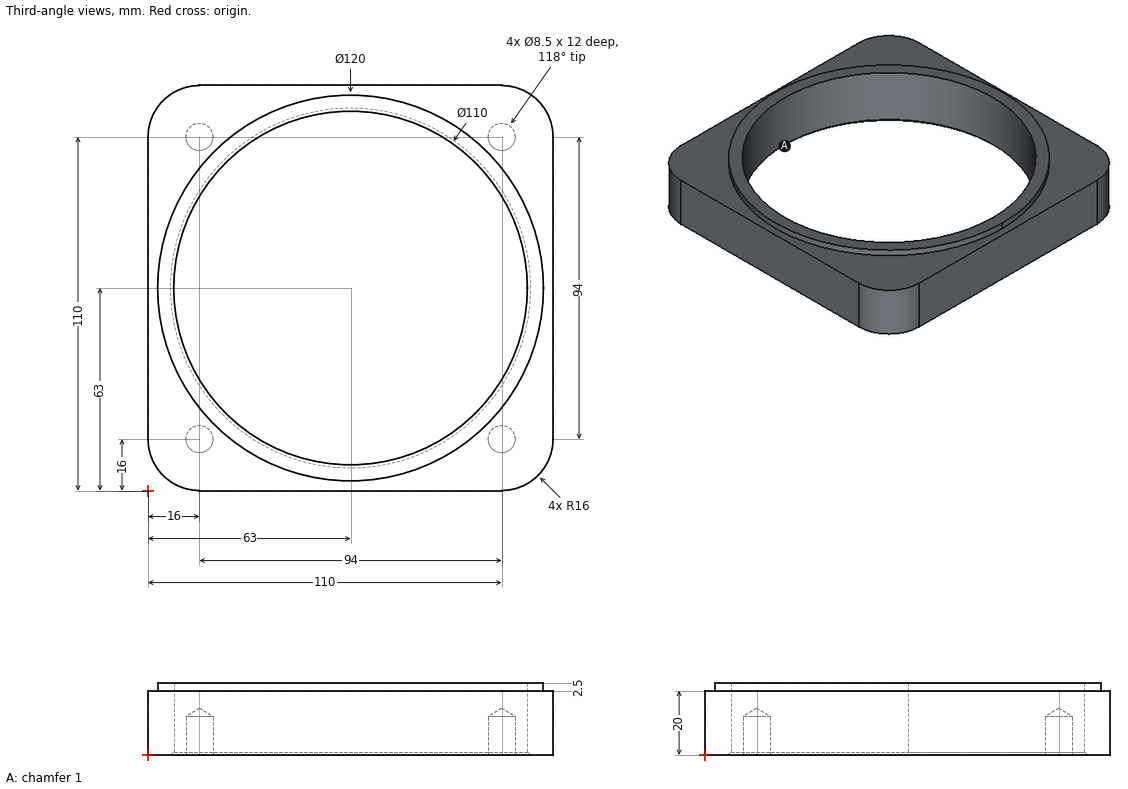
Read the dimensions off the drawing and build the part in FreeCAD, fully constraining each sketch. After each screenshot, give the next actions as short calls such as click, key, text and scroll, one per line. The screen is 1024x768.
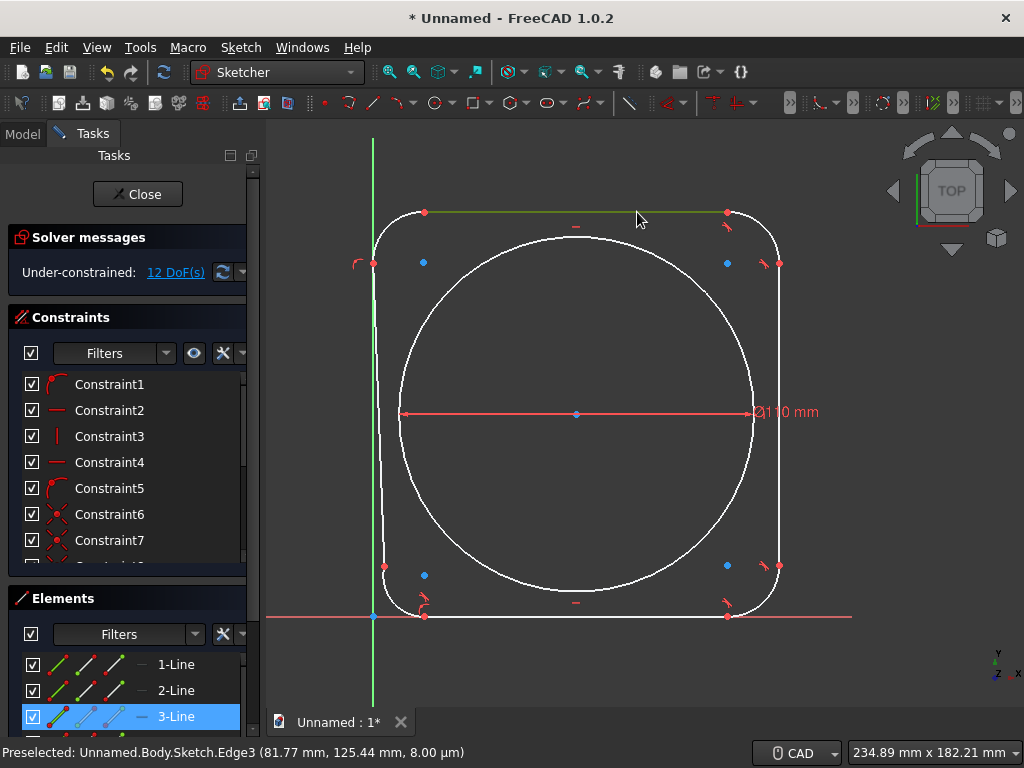
click(401, 217)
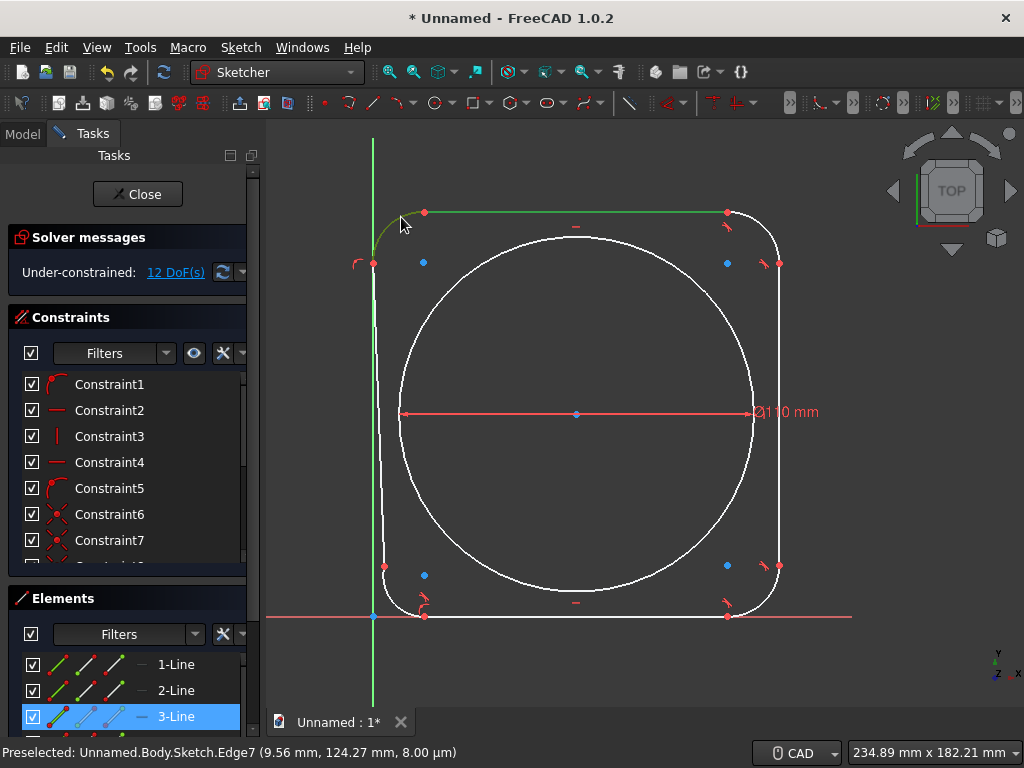
key(t)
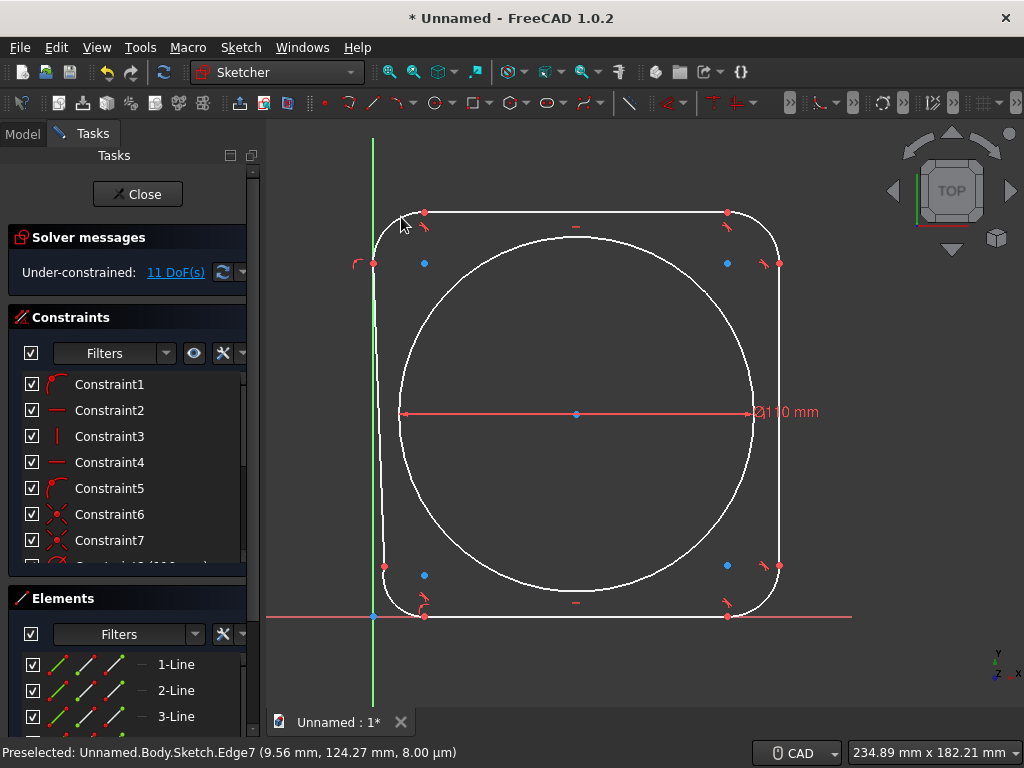
click(377, 354)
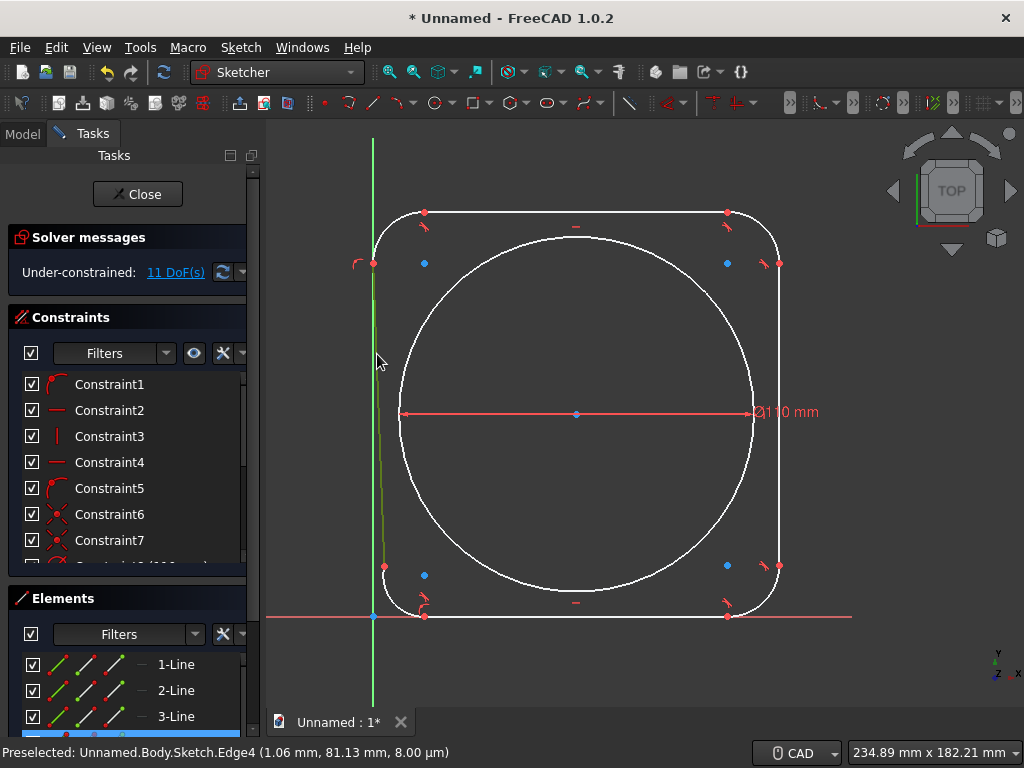
click(401, 218)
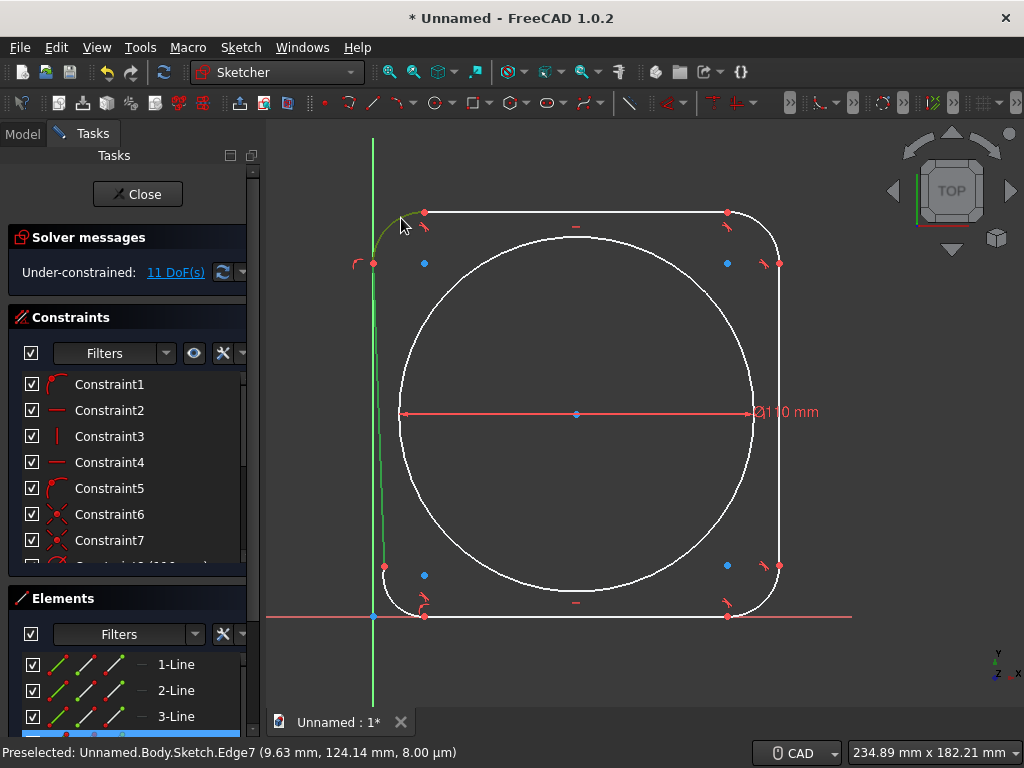
key(t)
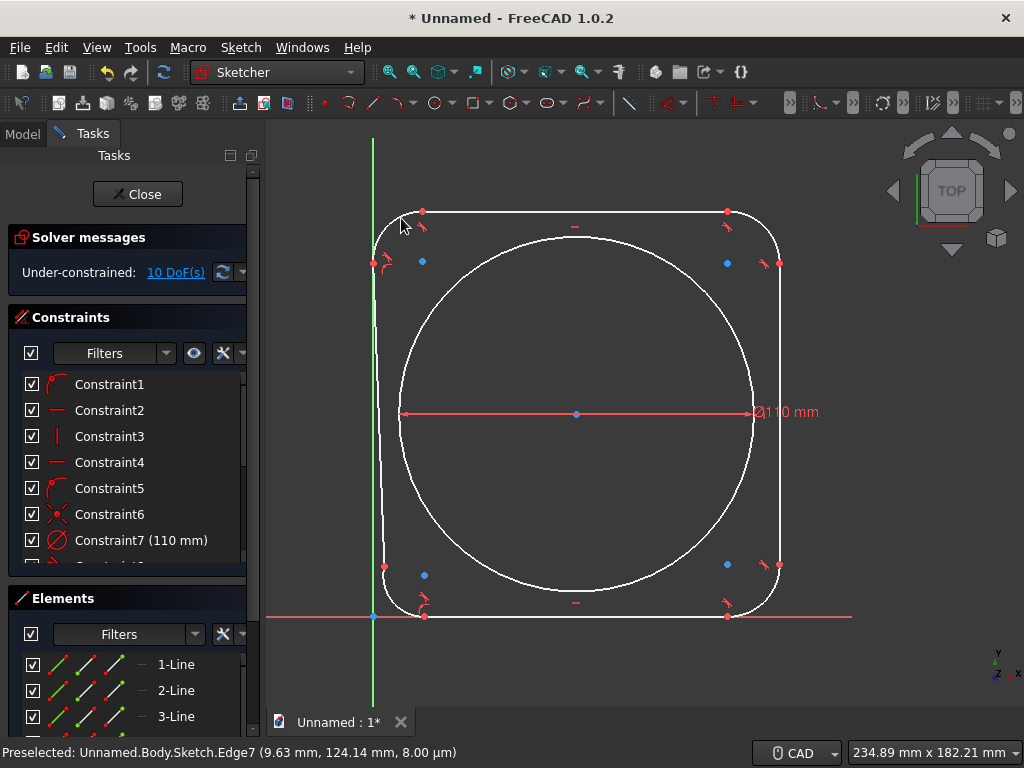
click(377, 354)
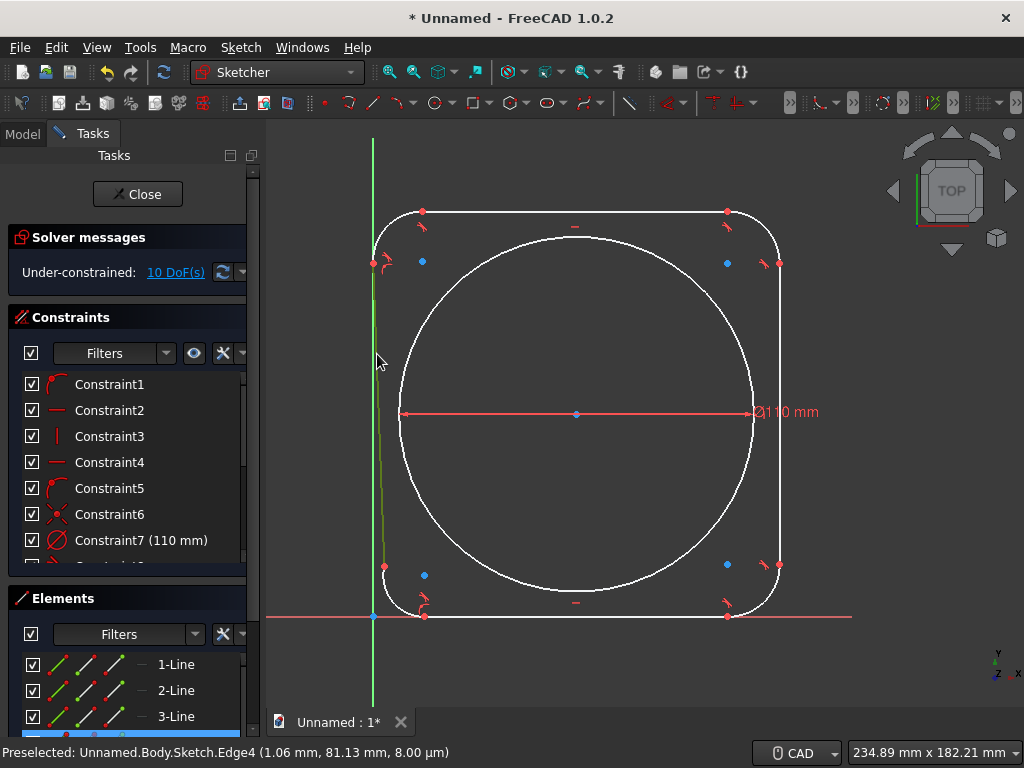
click(385, 588)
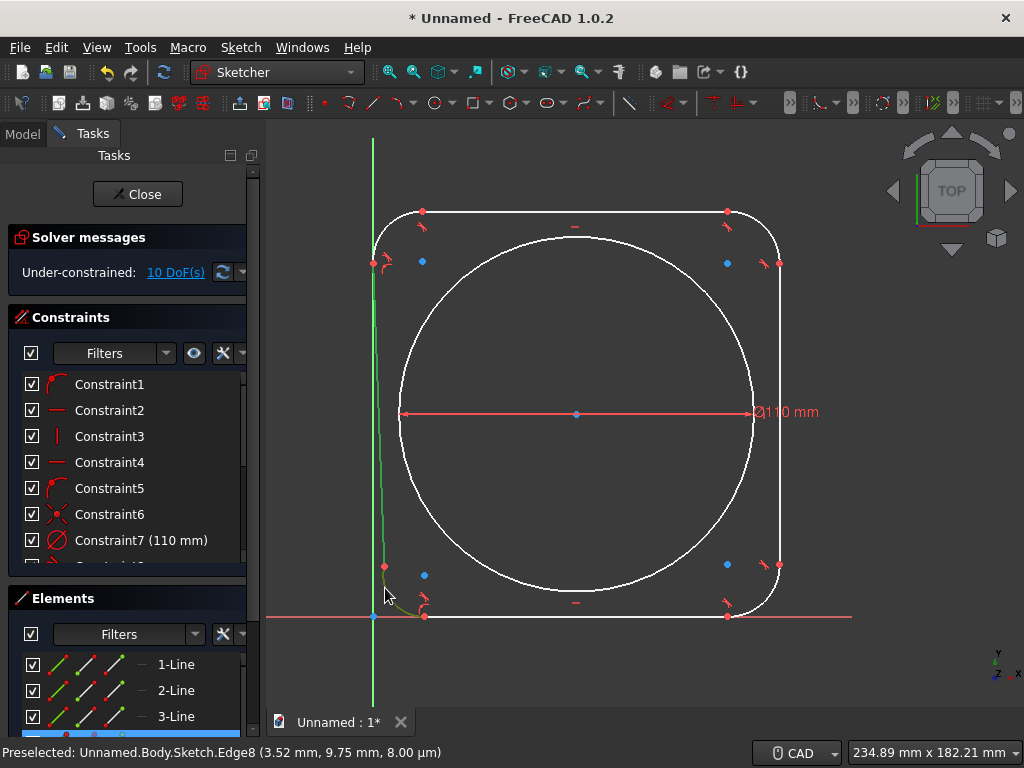
key(t)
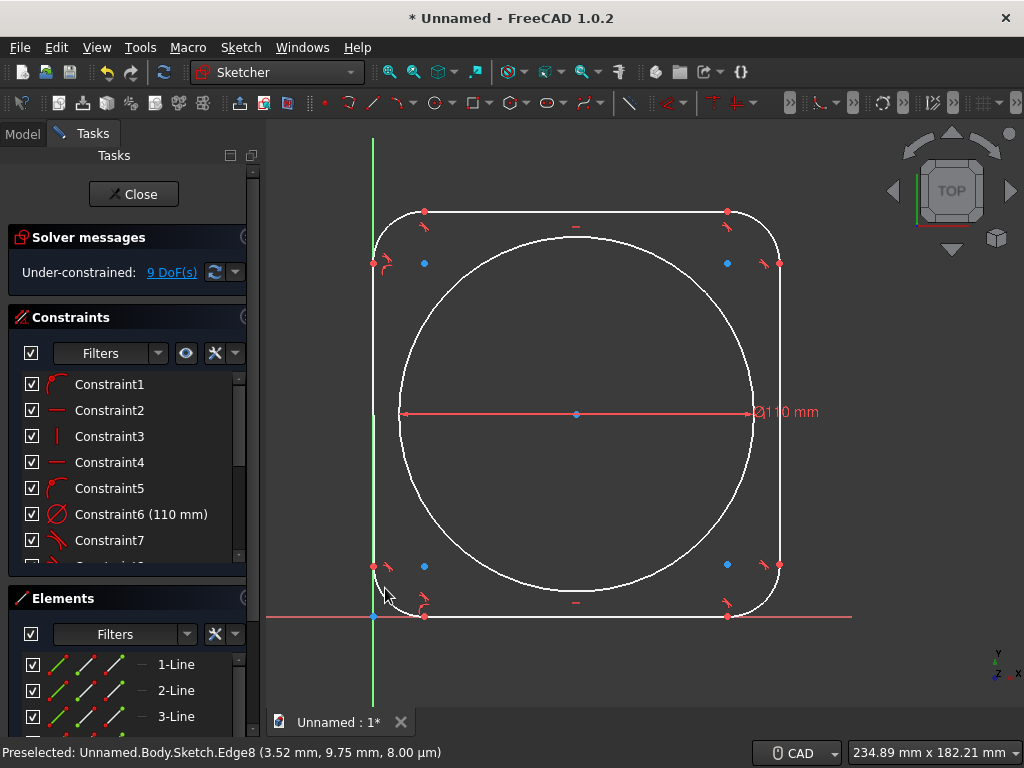
click(373, 354)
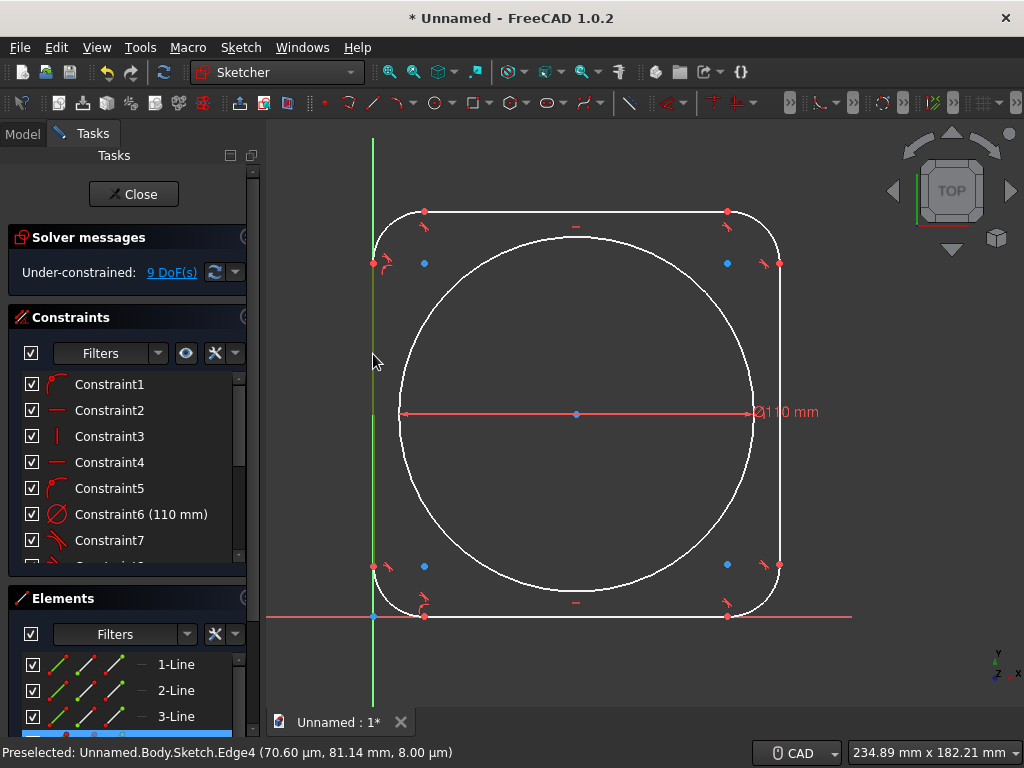
click(756, 104)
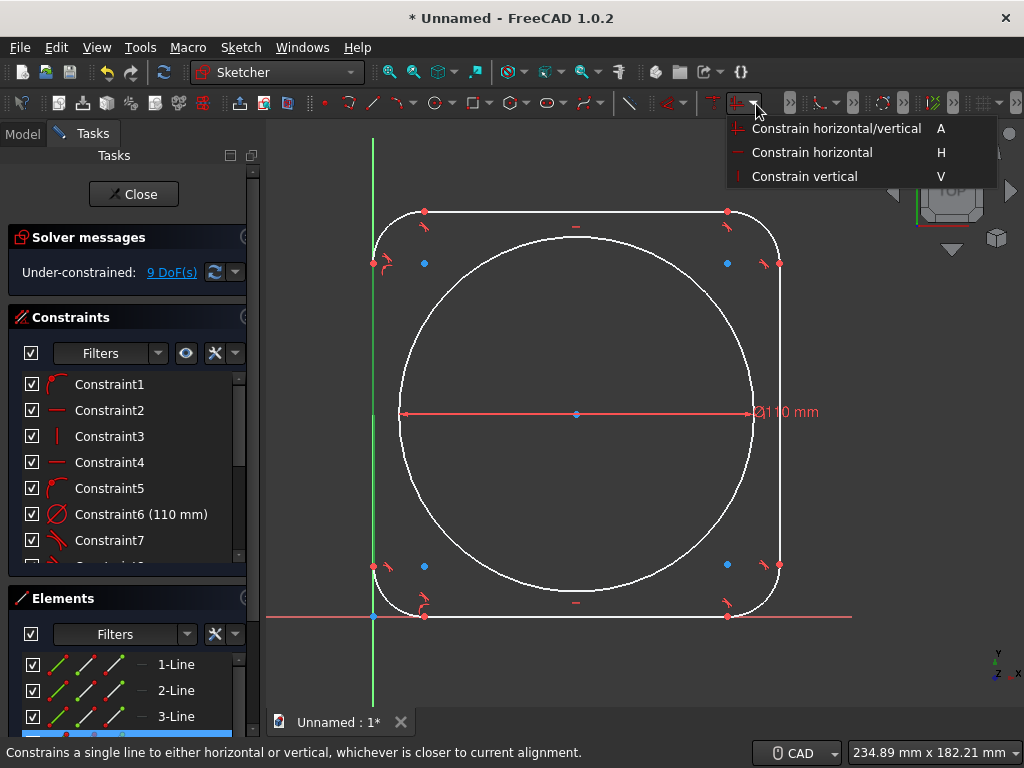
click(862, 176)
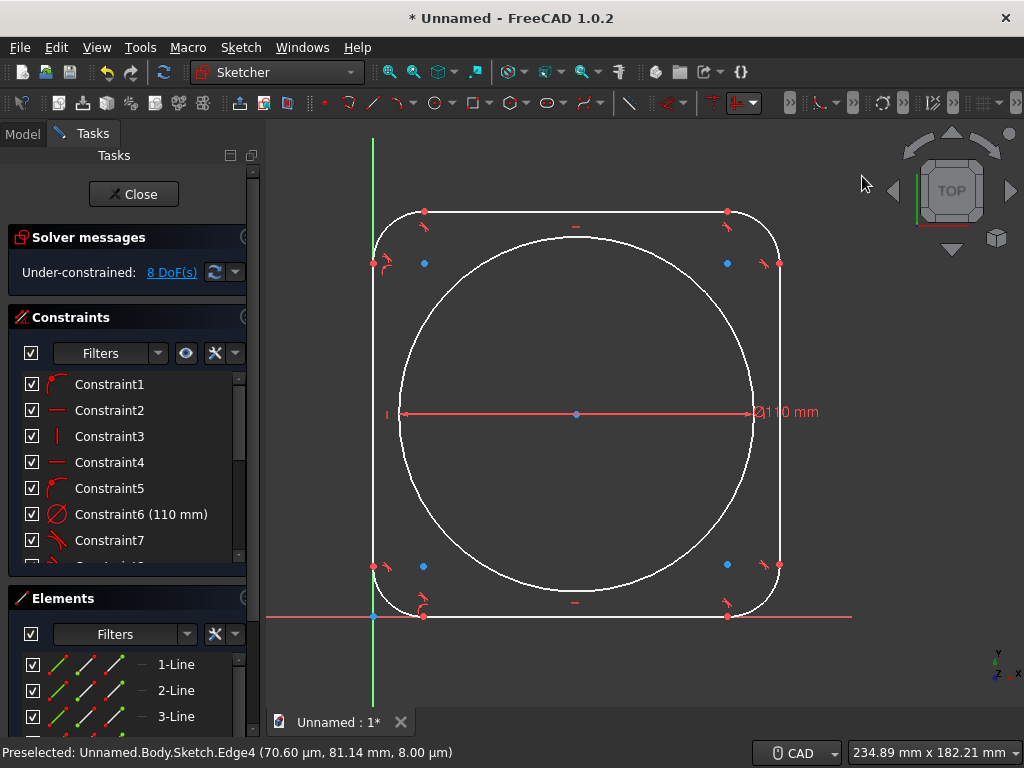
click(774, 589)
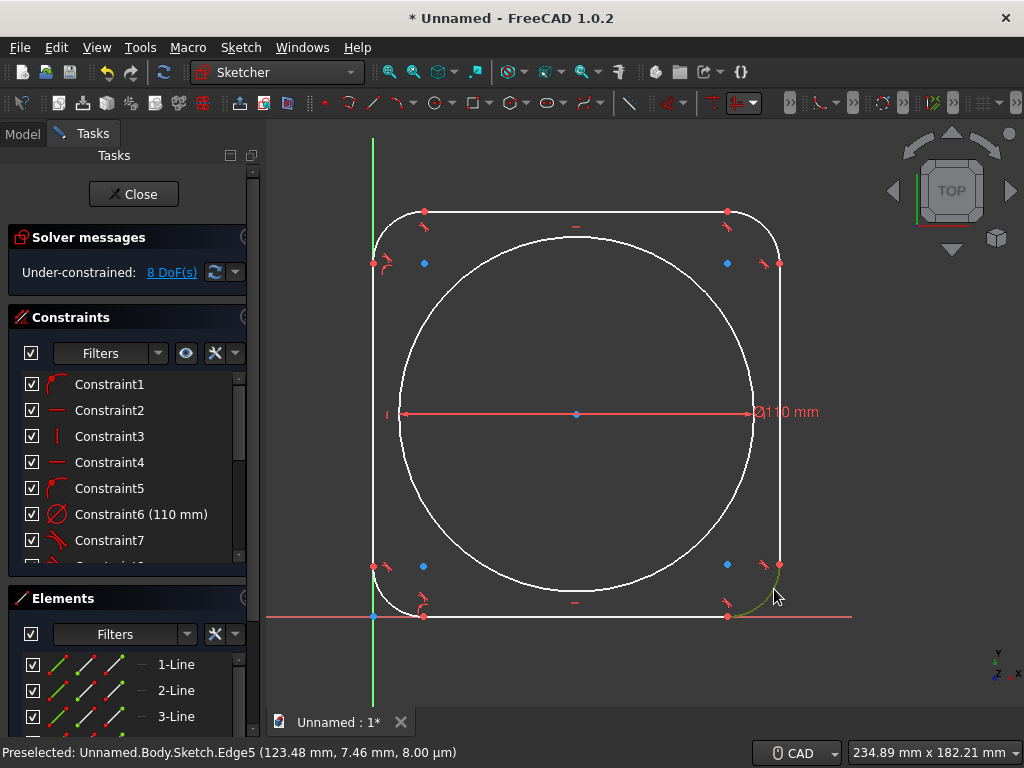
click(774, 240)